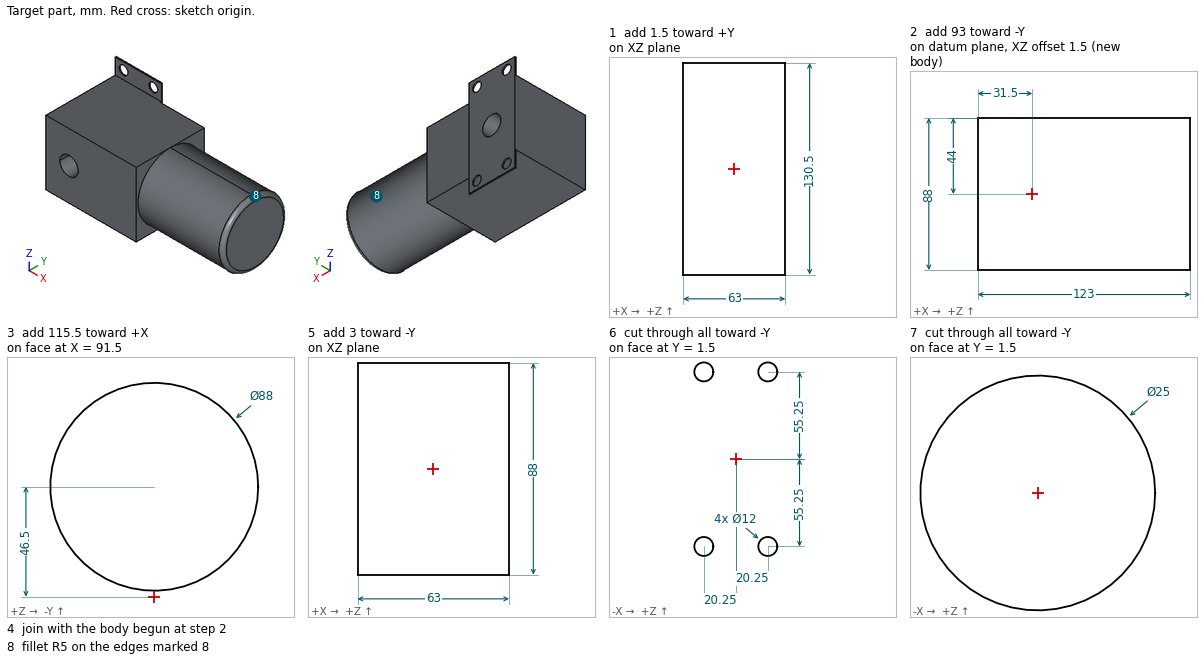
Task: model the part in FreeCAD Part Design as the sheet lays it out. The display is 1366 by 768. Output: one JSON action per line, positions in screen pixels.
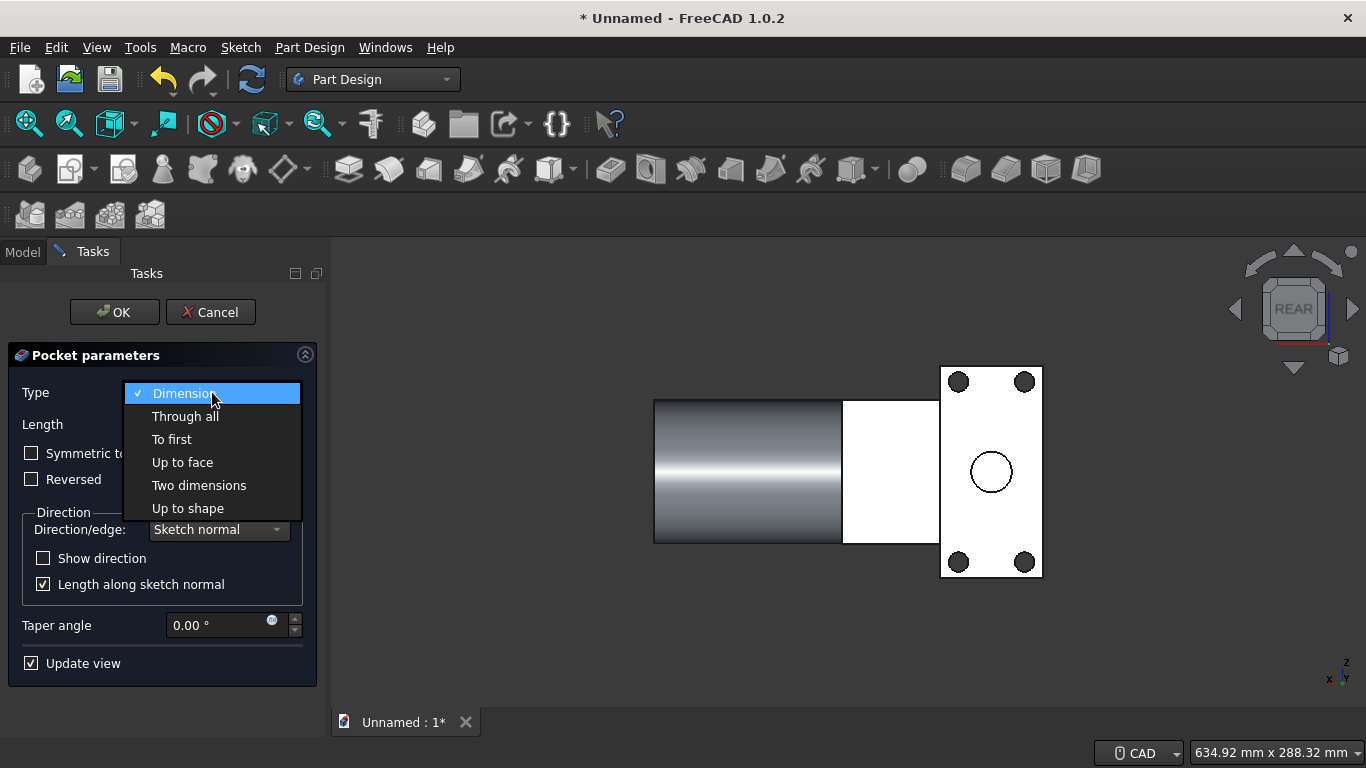
{"action": "left_click", "coordinate": [212, 416]}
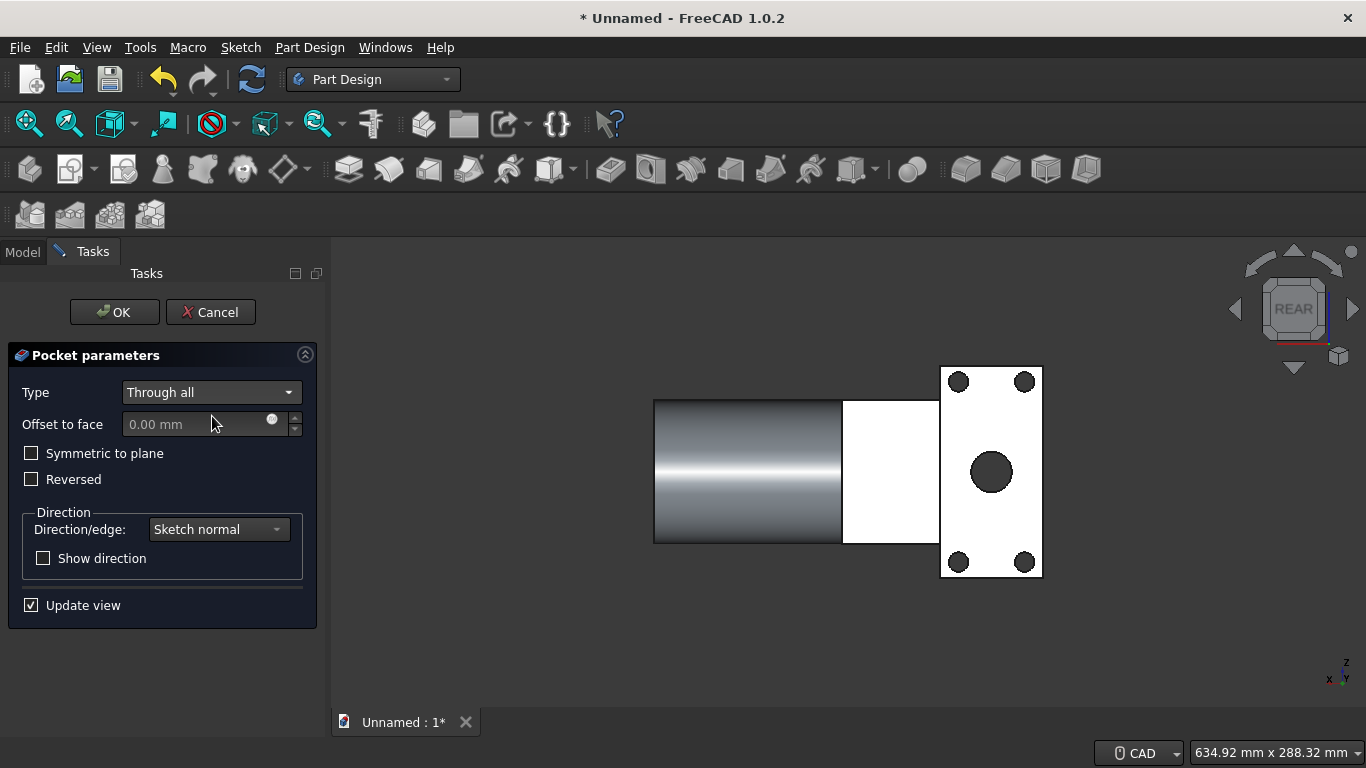
{"action": "left_click", "coordinate": [115, 312]}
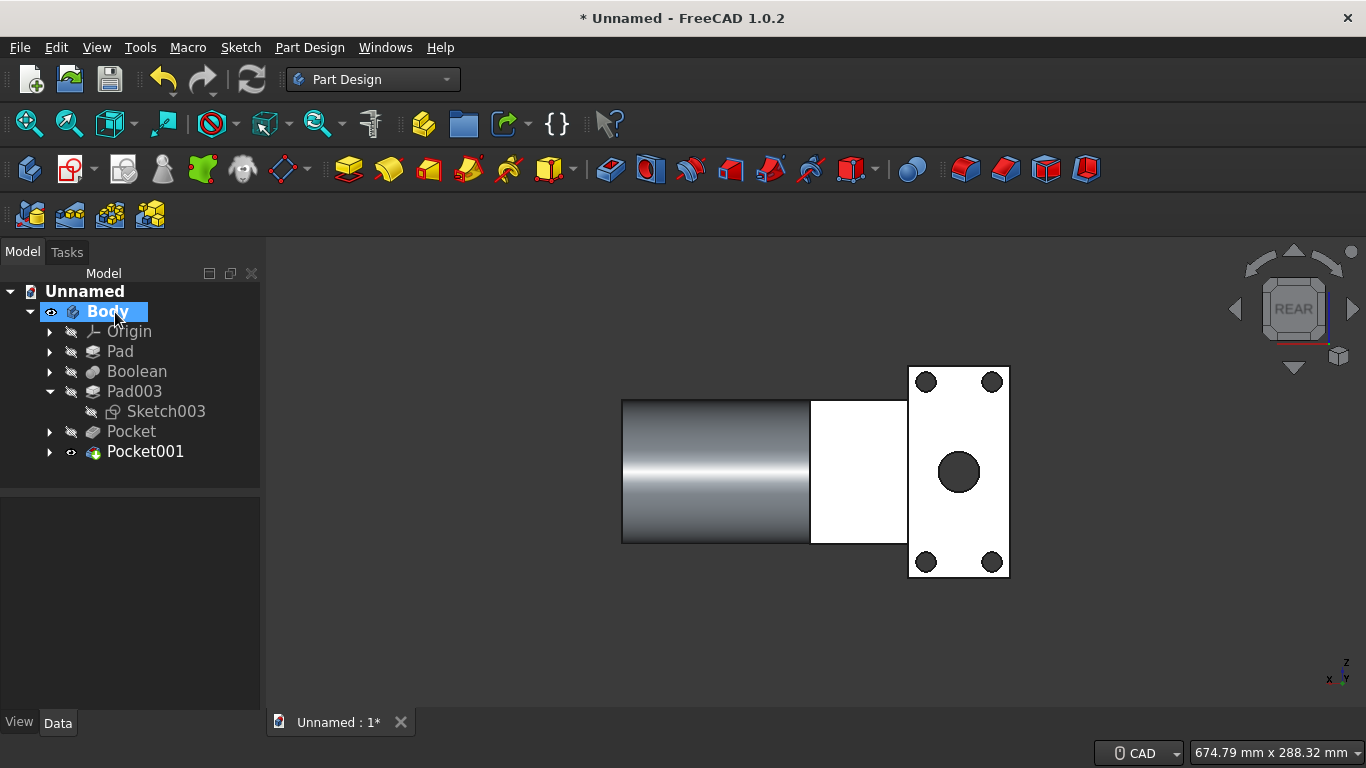
{"action": "left_click", "coordinate": [622, 419]}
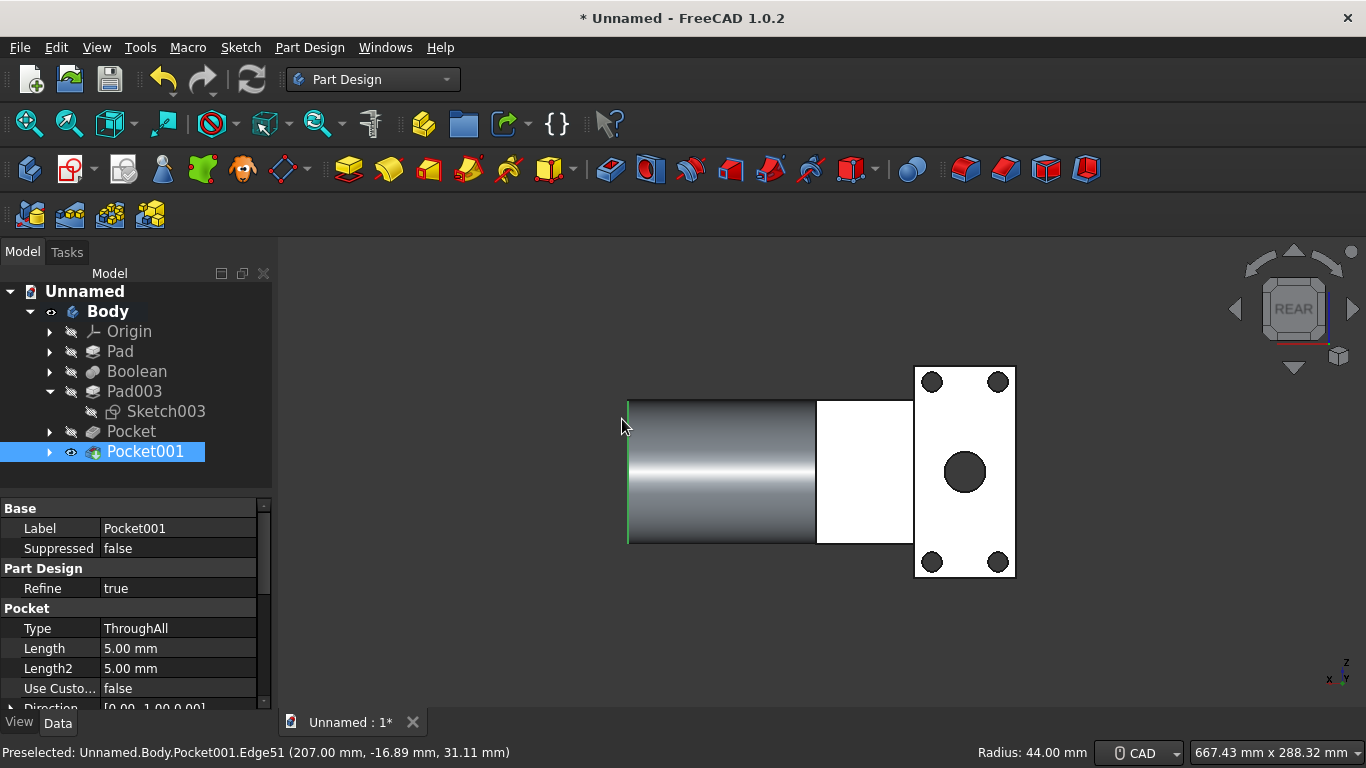
{"action": "left_click", "coordinate": [966, 170]}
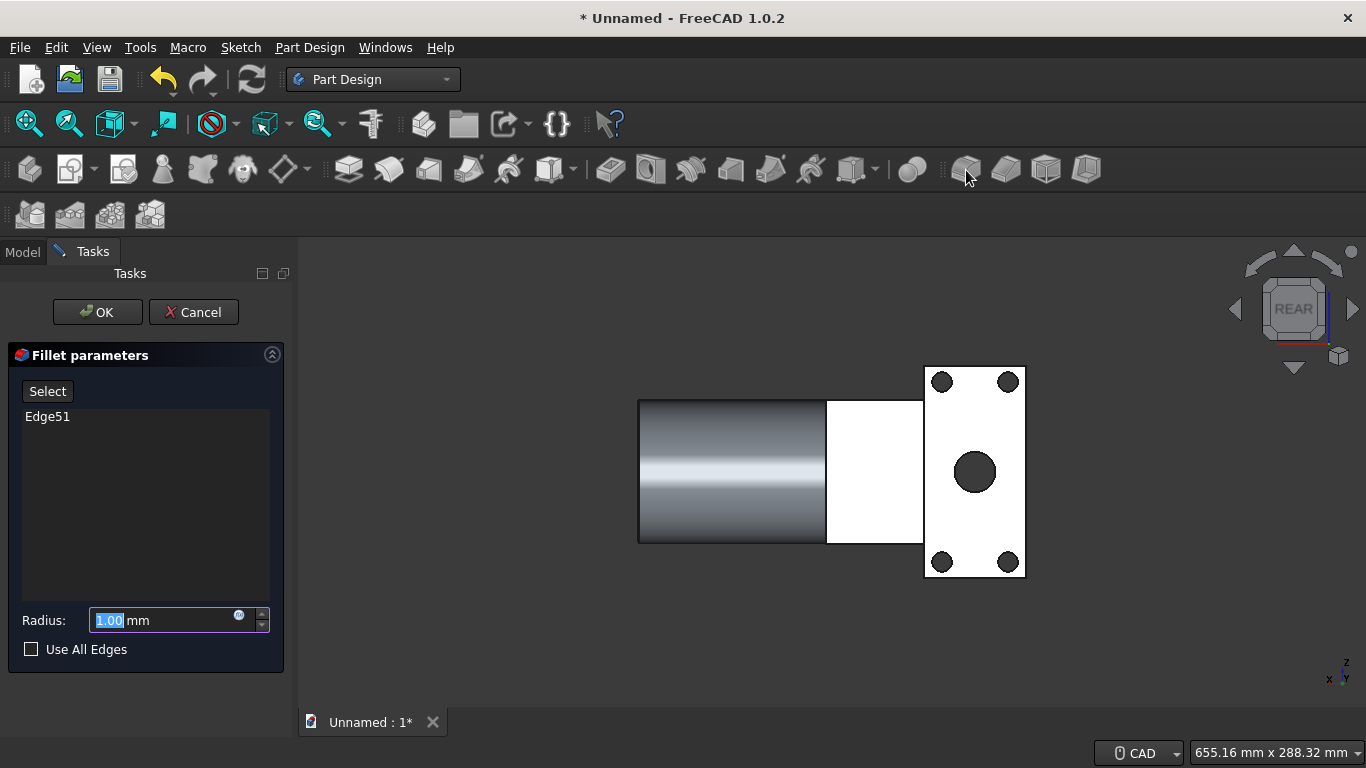
{"action": "type", "text": "5"}
{"action": "key", "text": "Tab"}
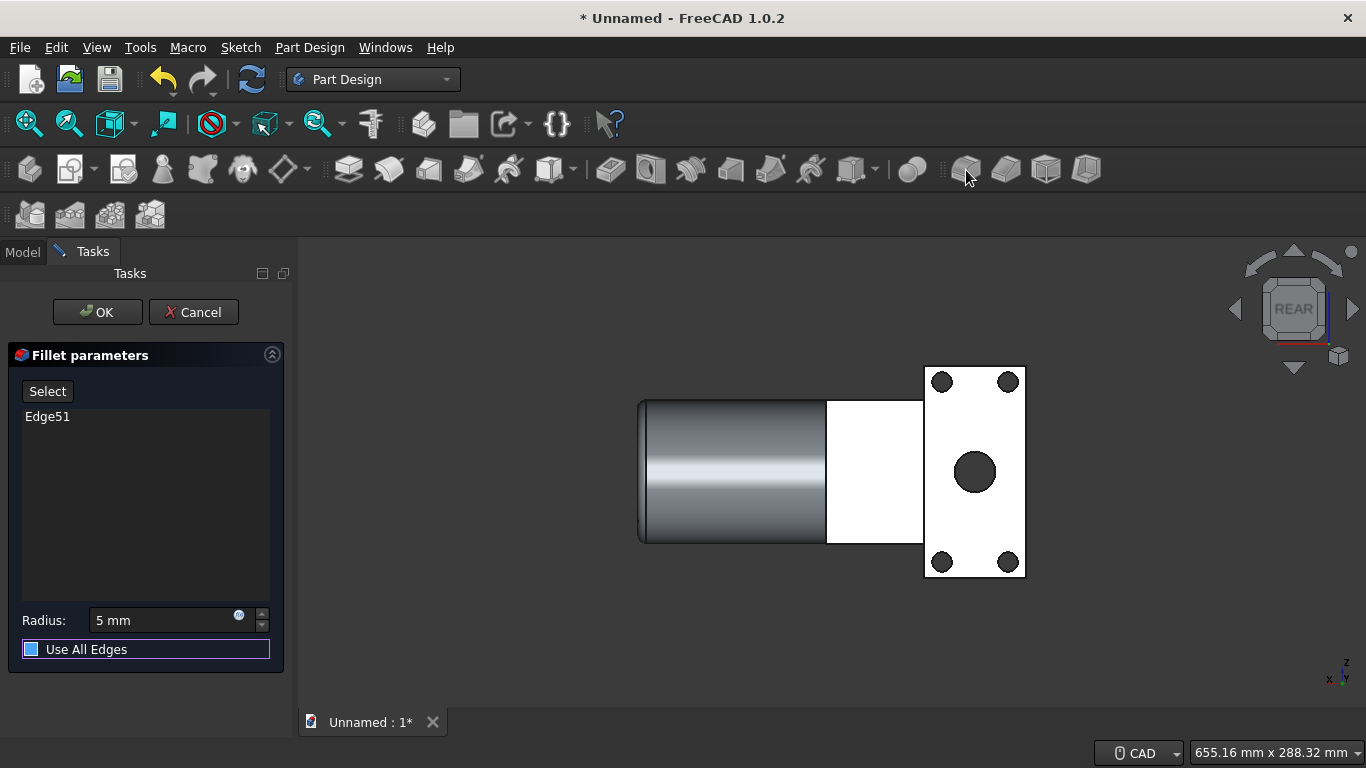
{"action": "left_click", "coordinate": [98, 312]}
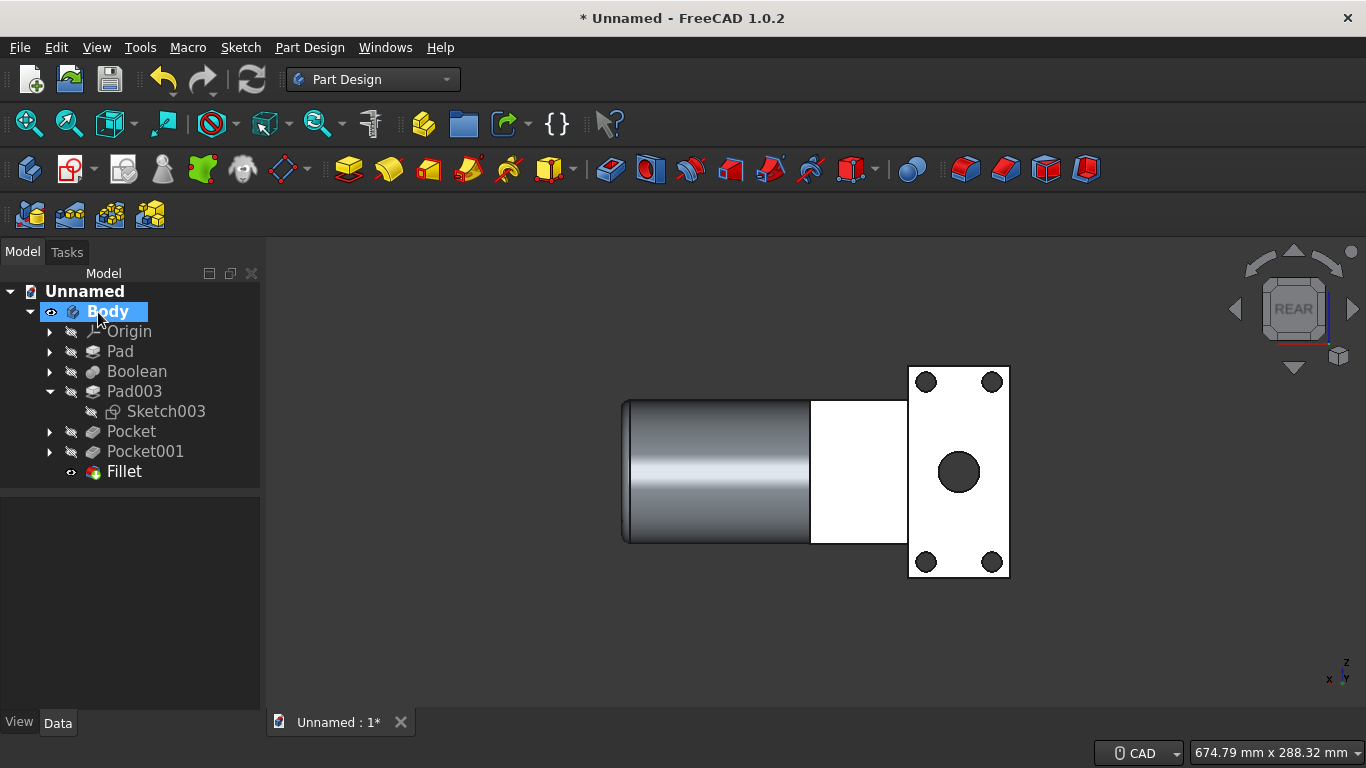
{"action": "key", "text": "0"}